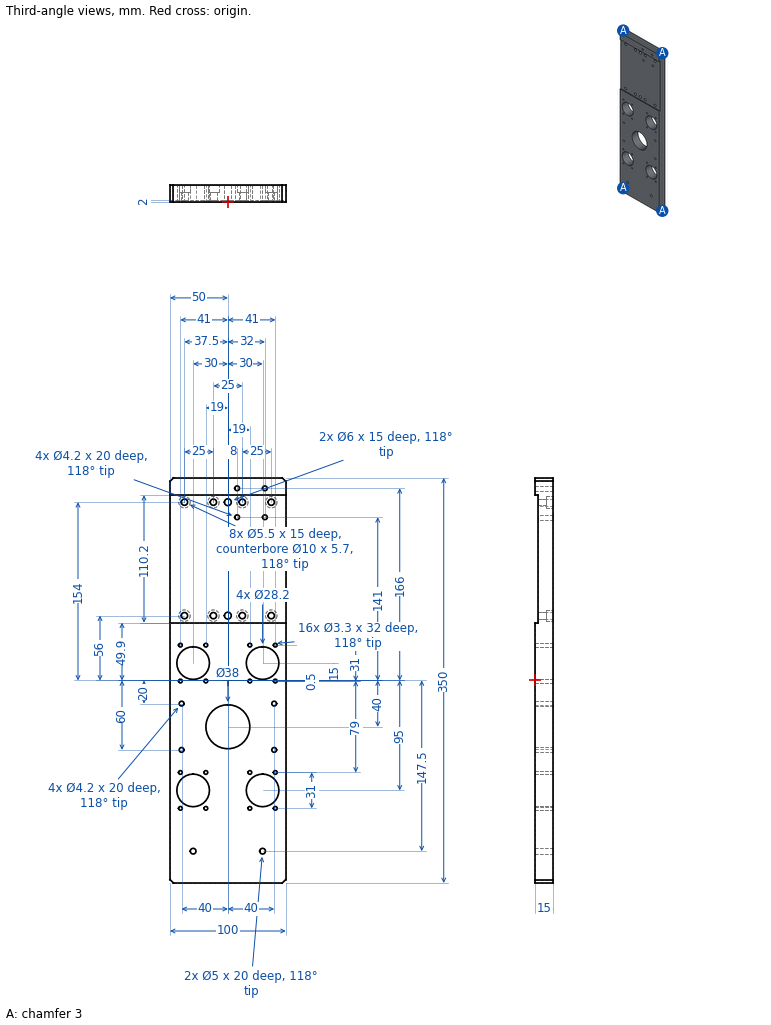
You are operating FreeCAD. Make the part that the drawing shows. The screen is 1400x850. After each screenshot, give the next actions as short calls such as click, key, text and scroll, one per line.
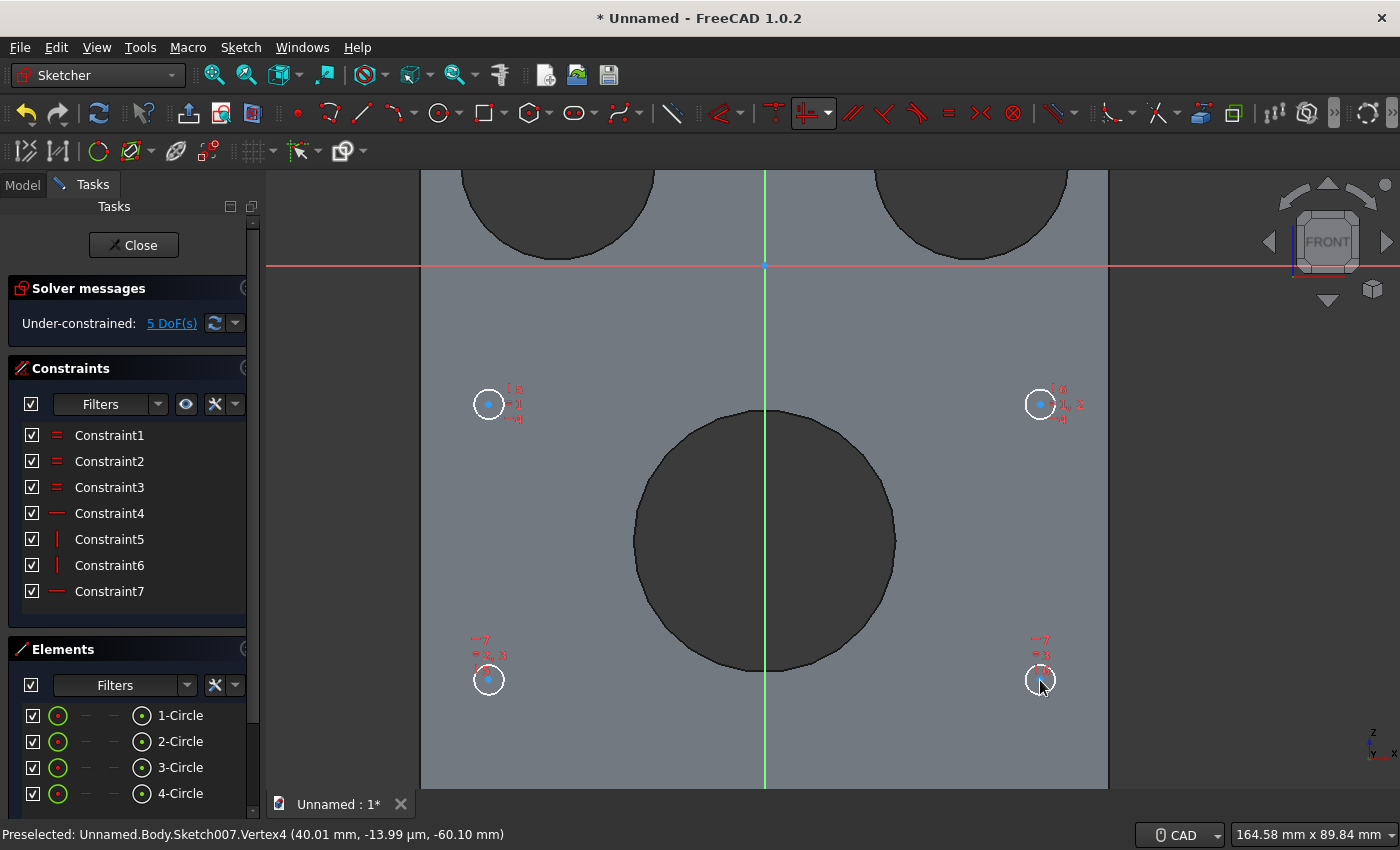
click(720, 114)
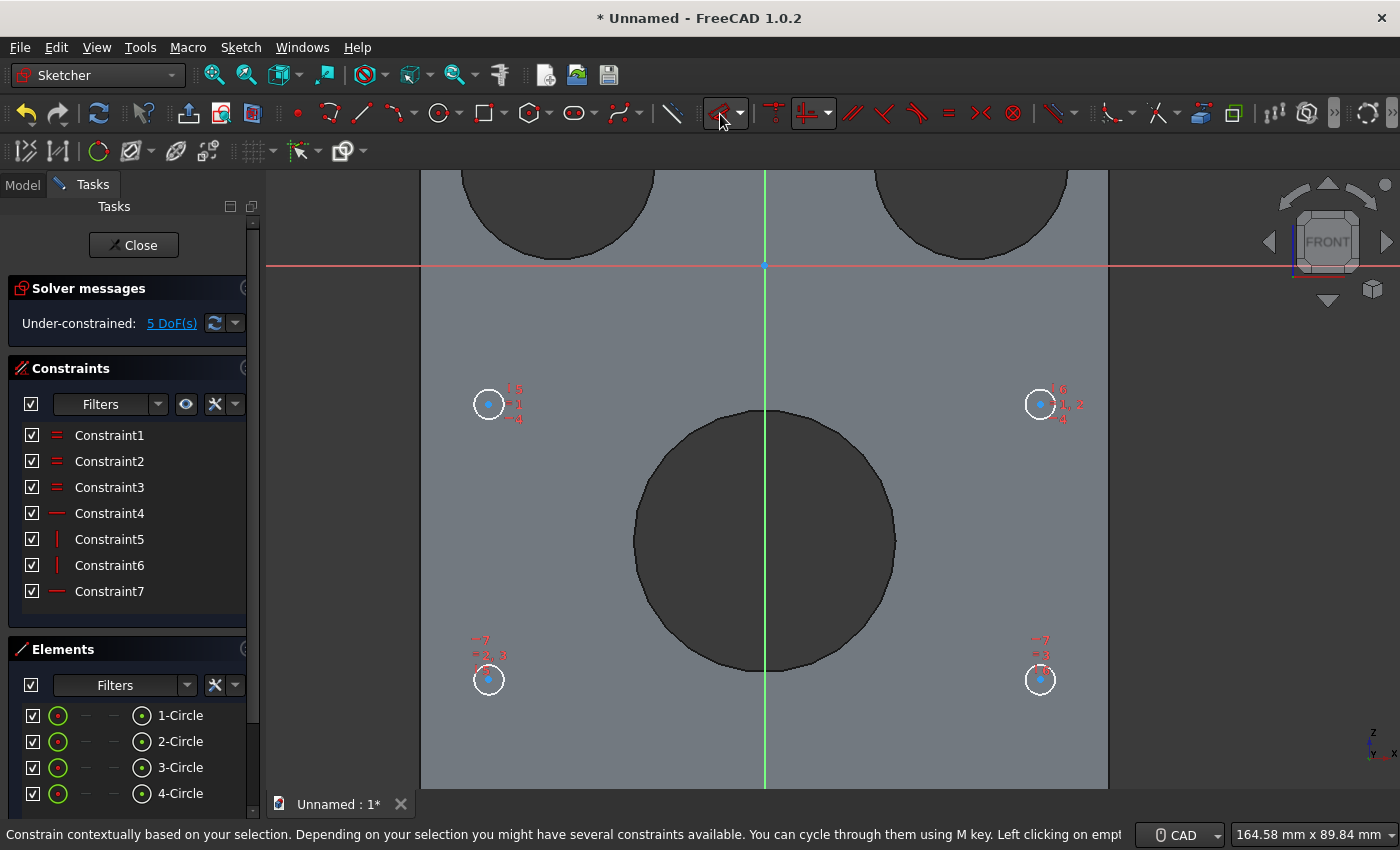
scroll(499, 394, up, 2)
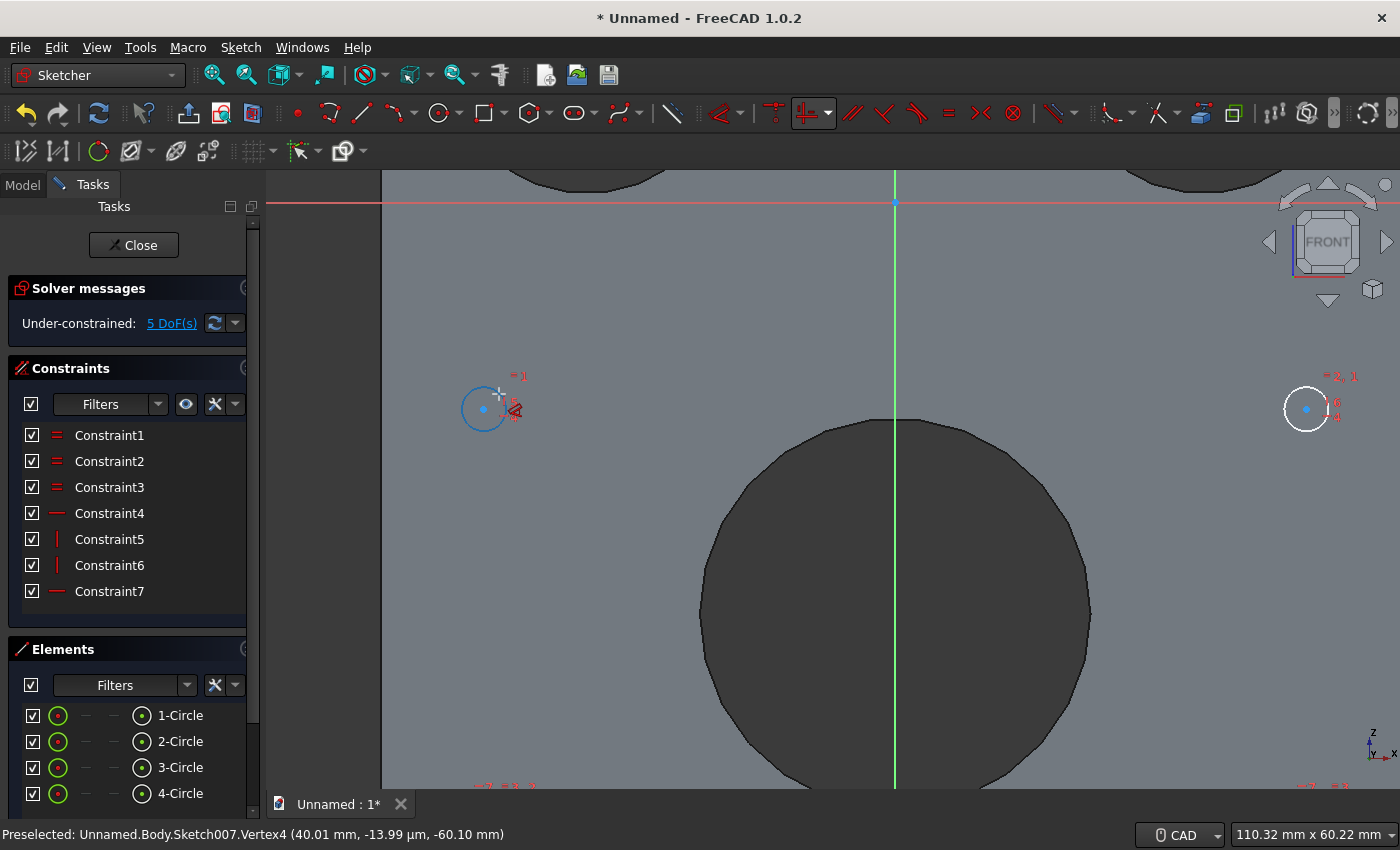
click(499, 394)
click(521, 371)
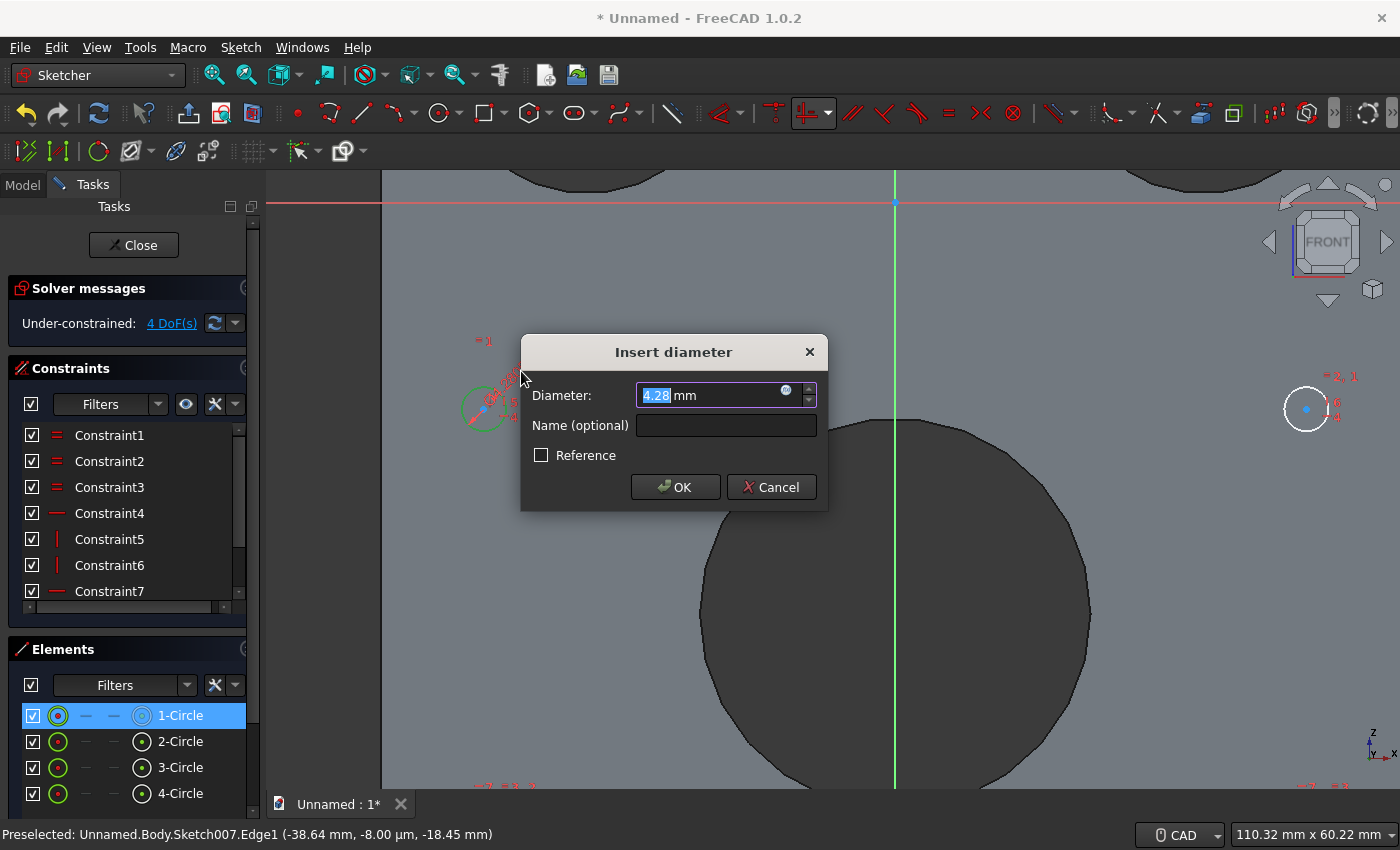
text(4.2)
key(Return)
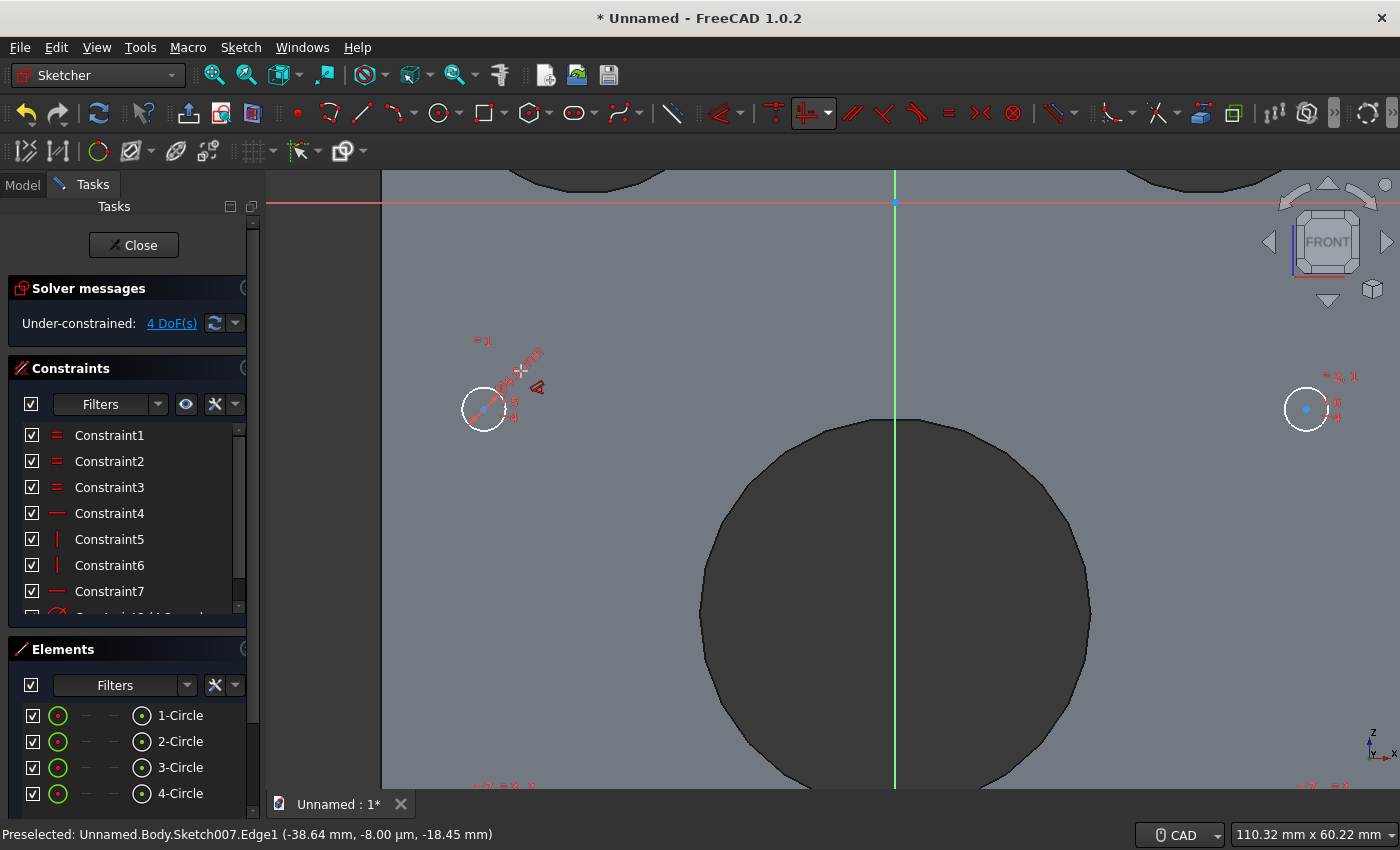
click(484, 409)
click(690, 443)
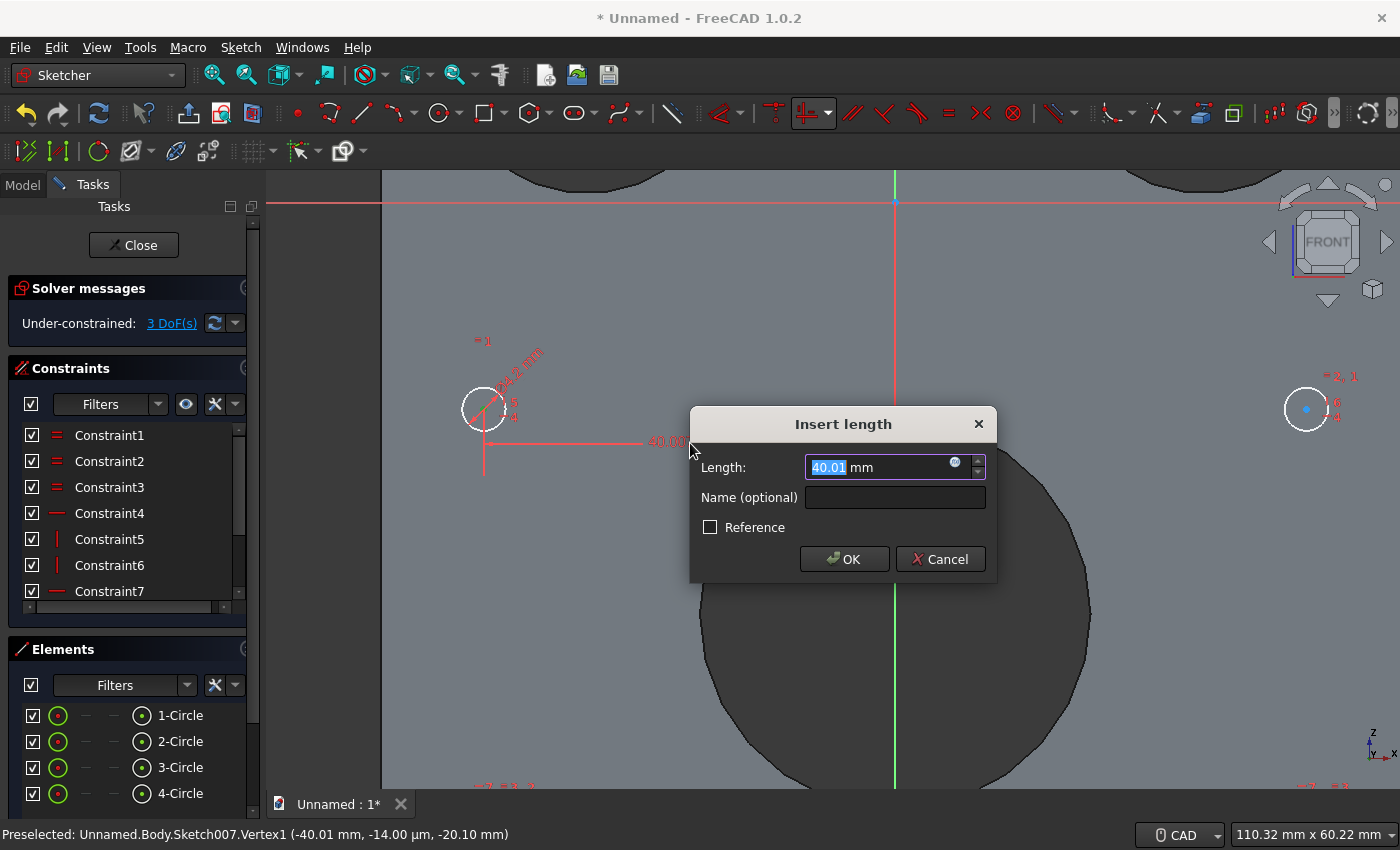
text(40)
key(Return)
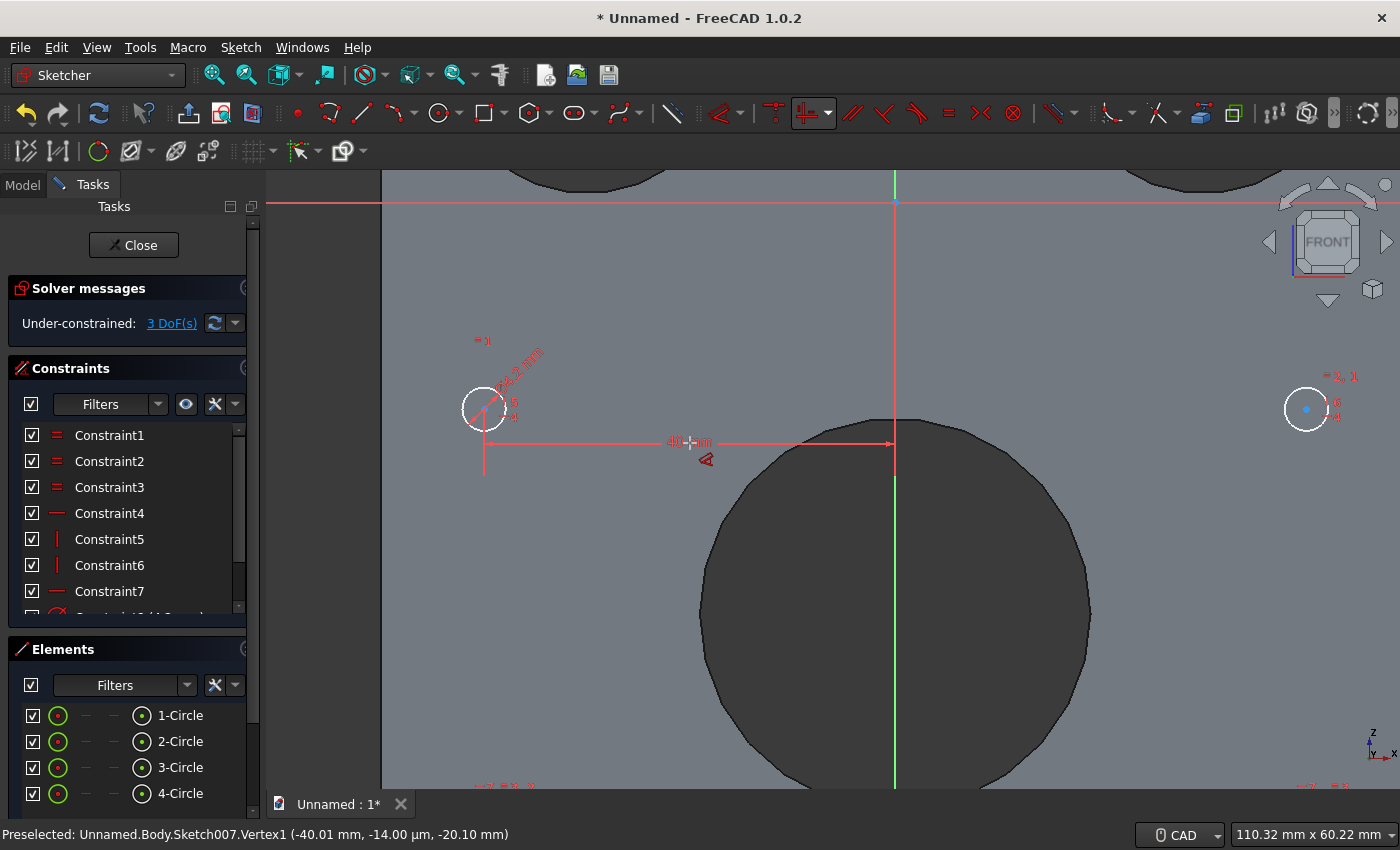
click(484, 409)
click(450, 306)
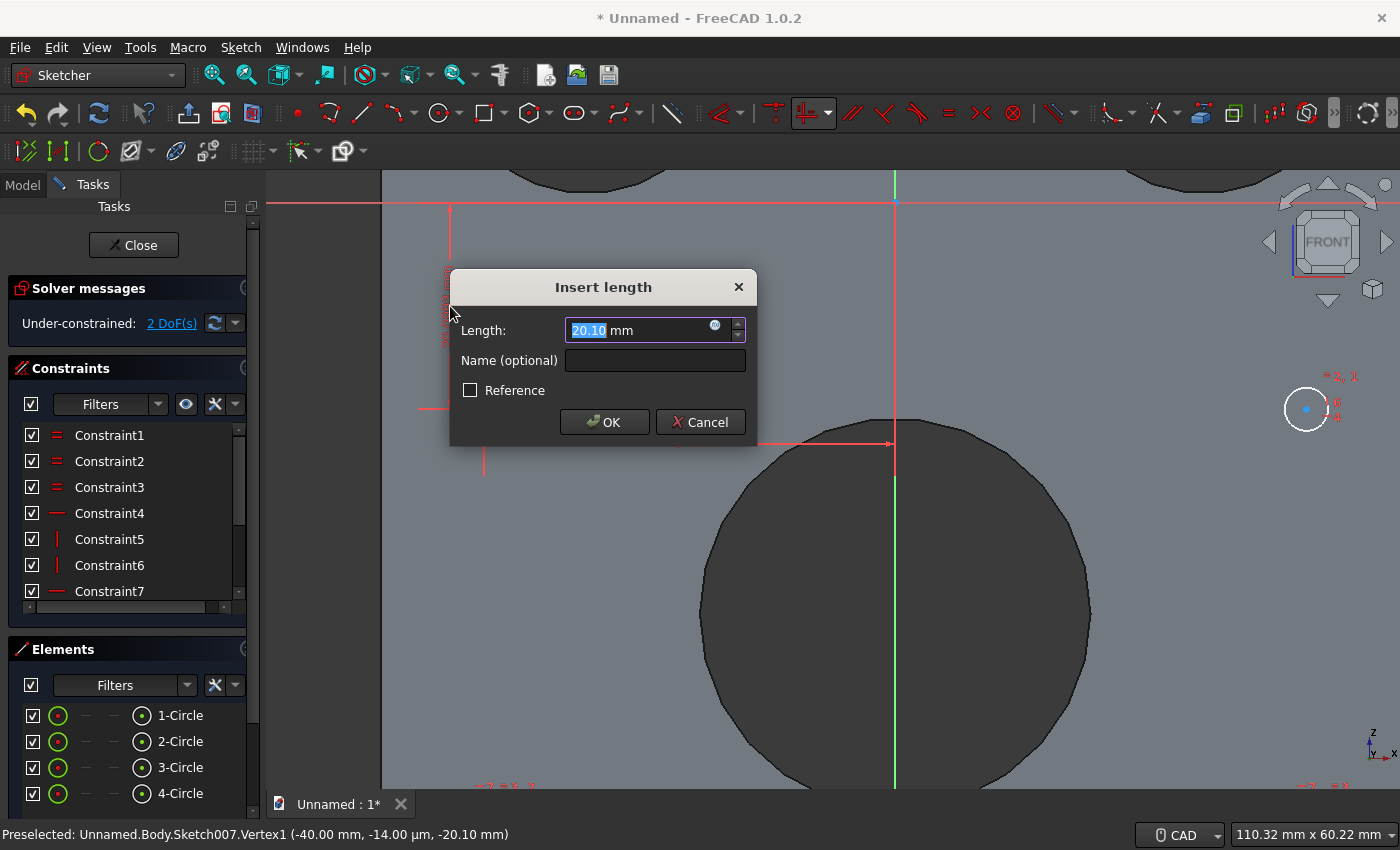
text(20)
key(Return)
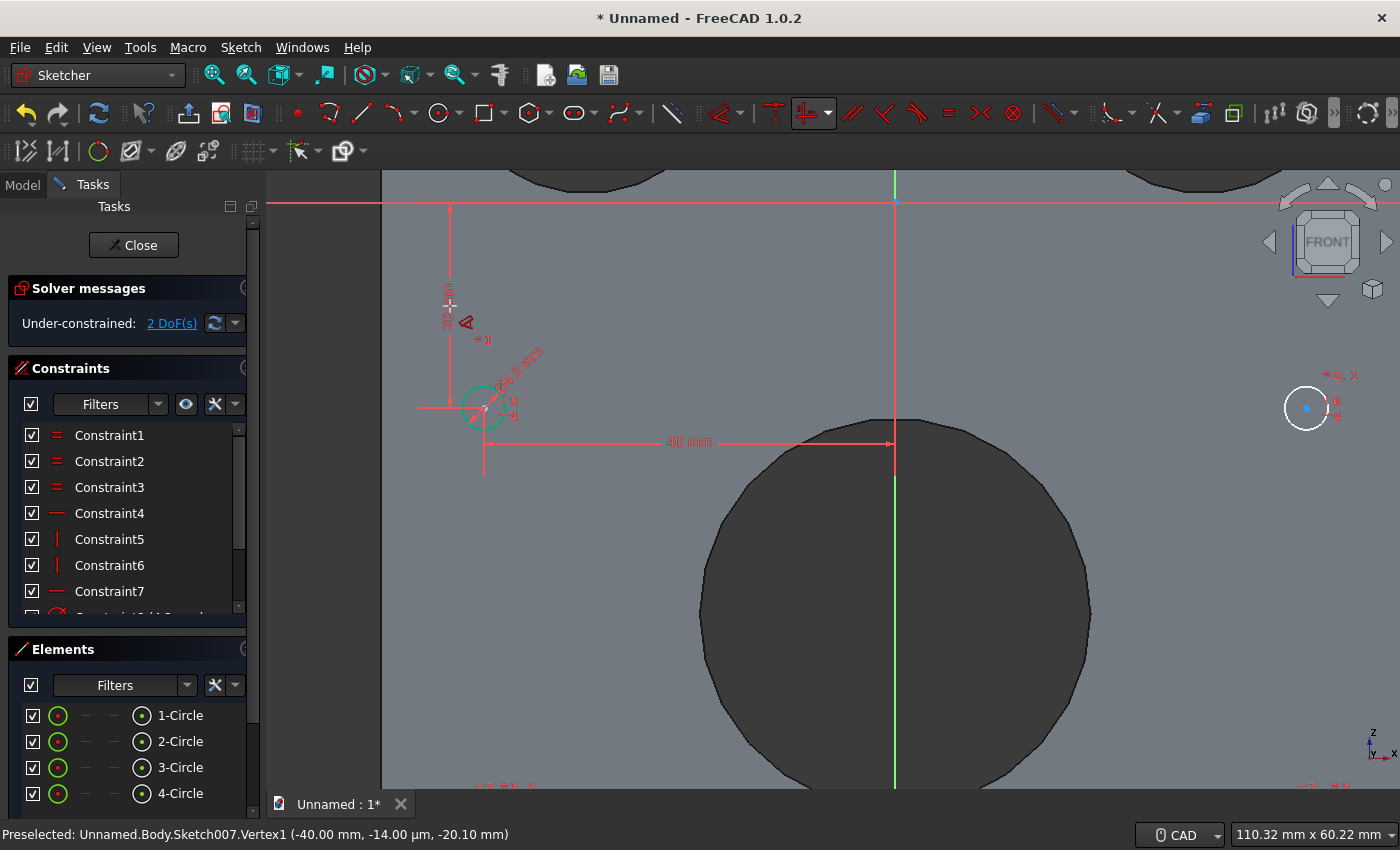
scroll(499, 394, down, 2)